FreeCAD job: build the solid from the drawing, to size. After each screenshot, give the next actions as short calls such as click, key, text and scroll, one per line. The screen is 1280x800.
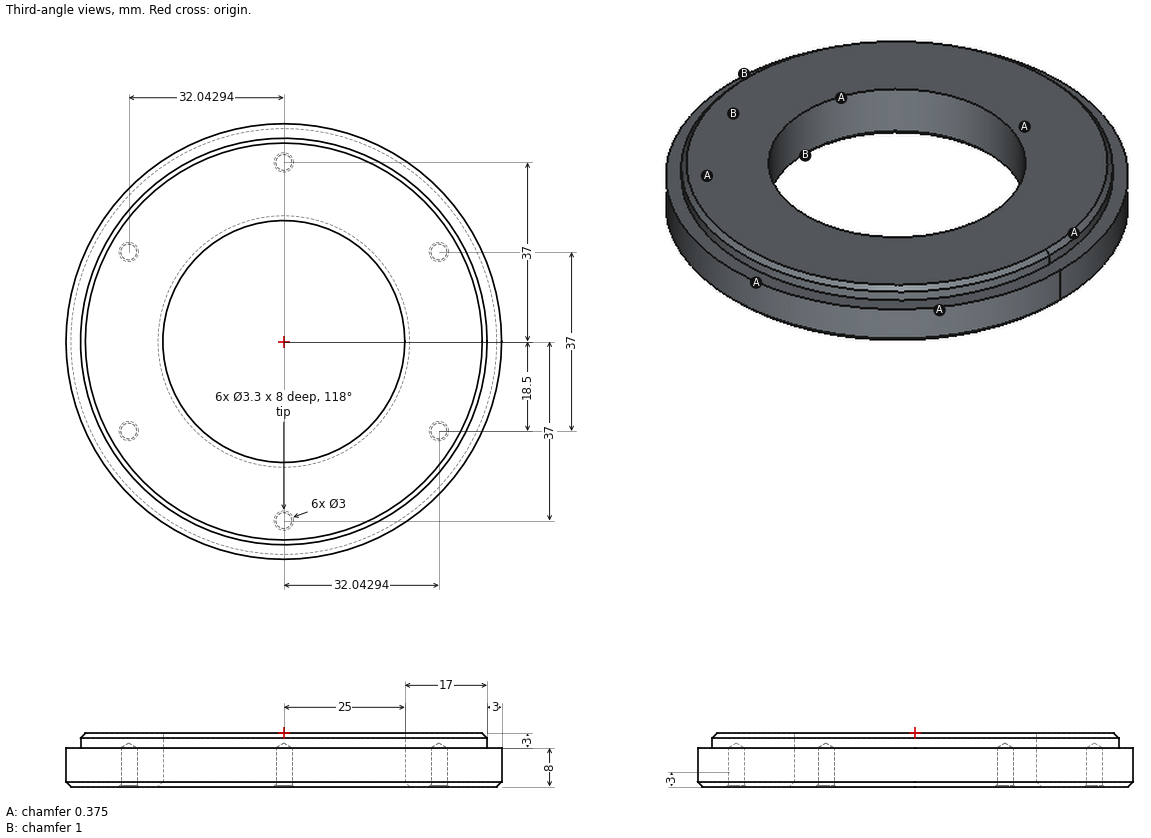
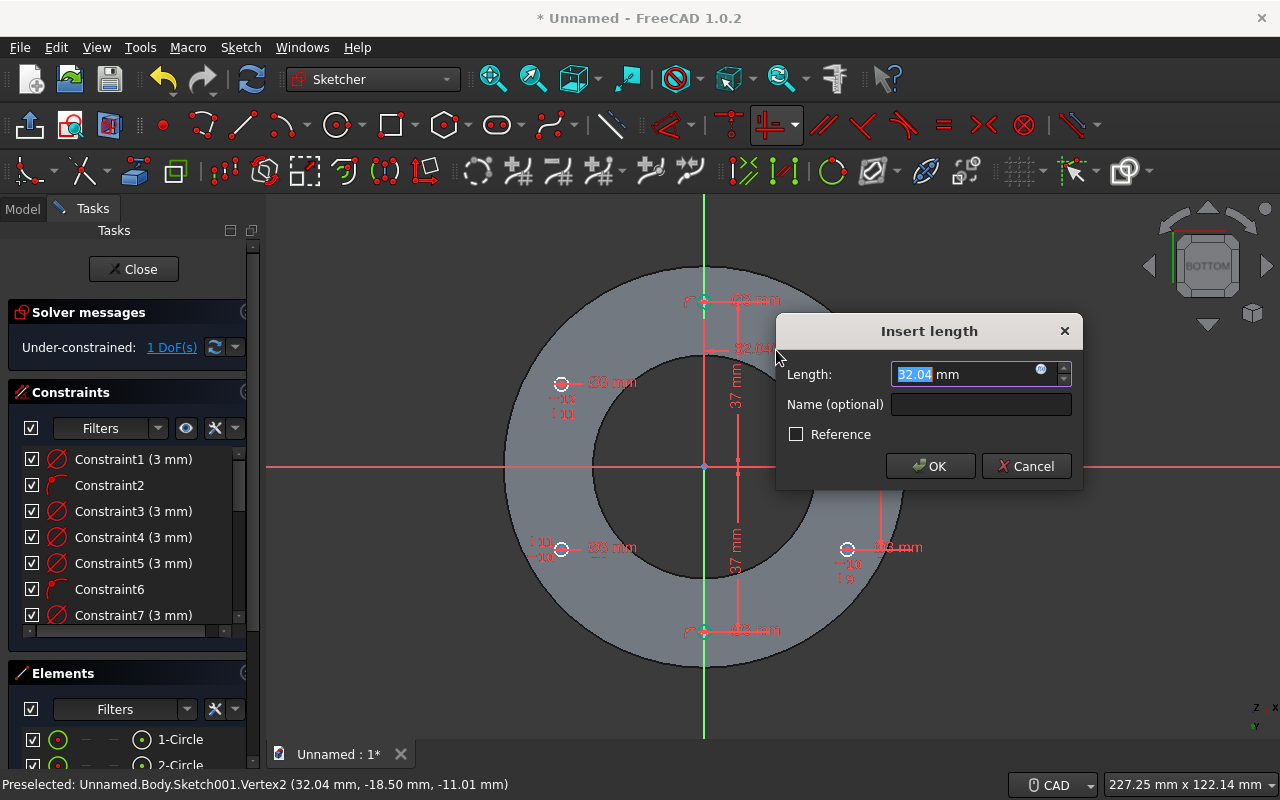
text(32.04294)
key(Return)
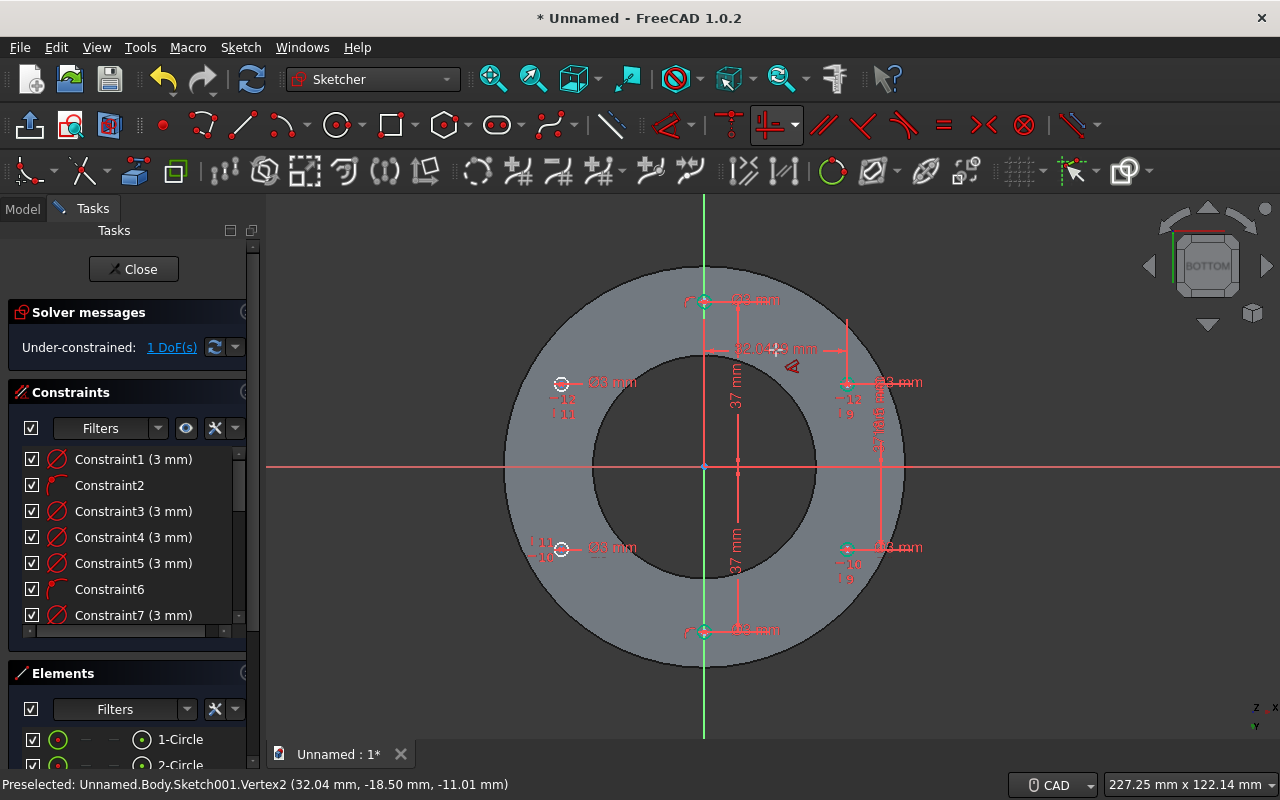
click(561, 550)
click(633, 584)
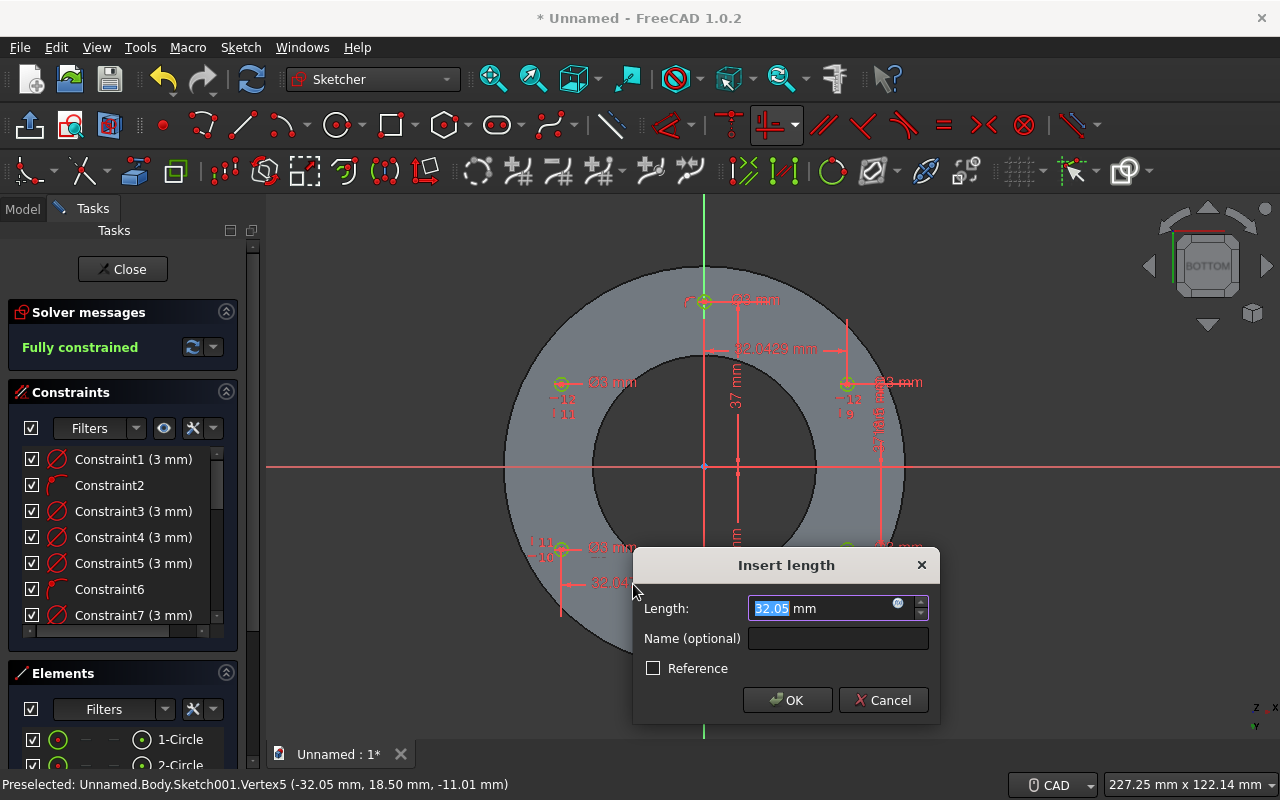
text(32.04294)
key(Return)
key(Escape)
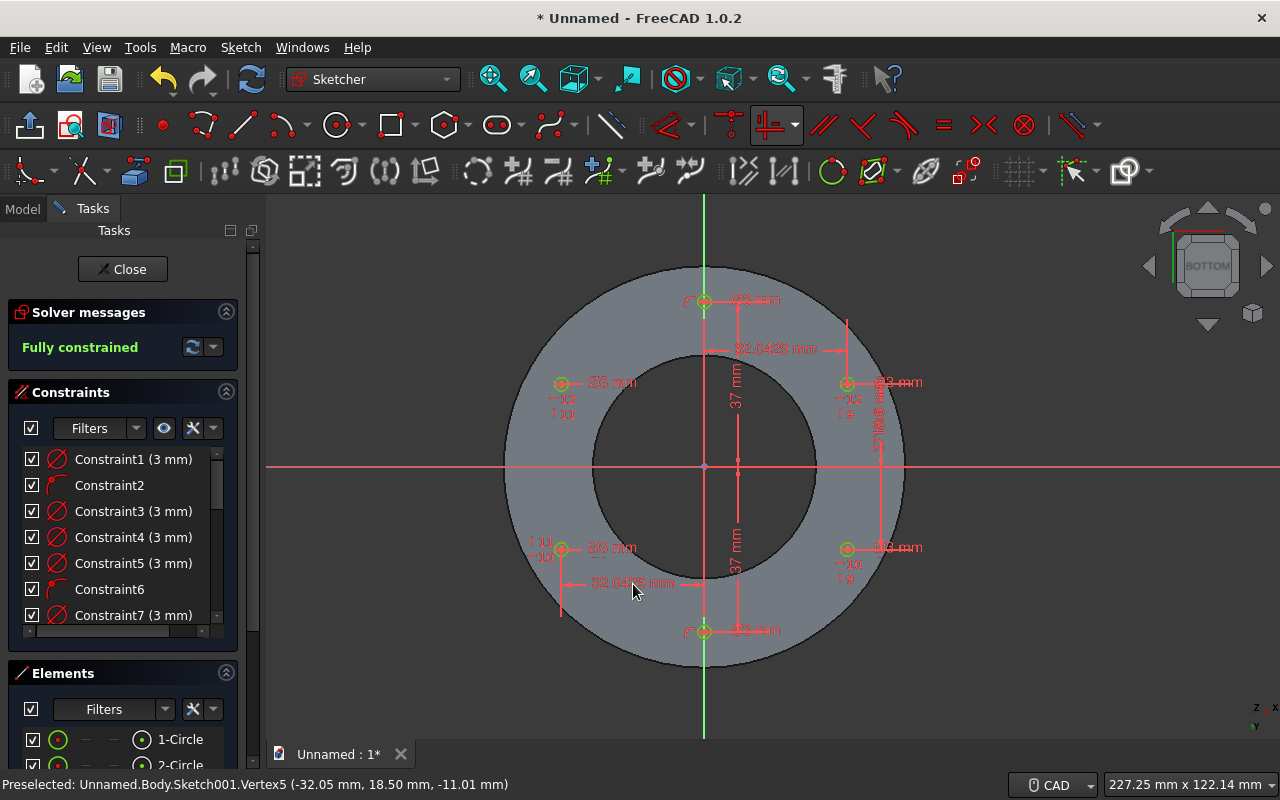
click(123, 269)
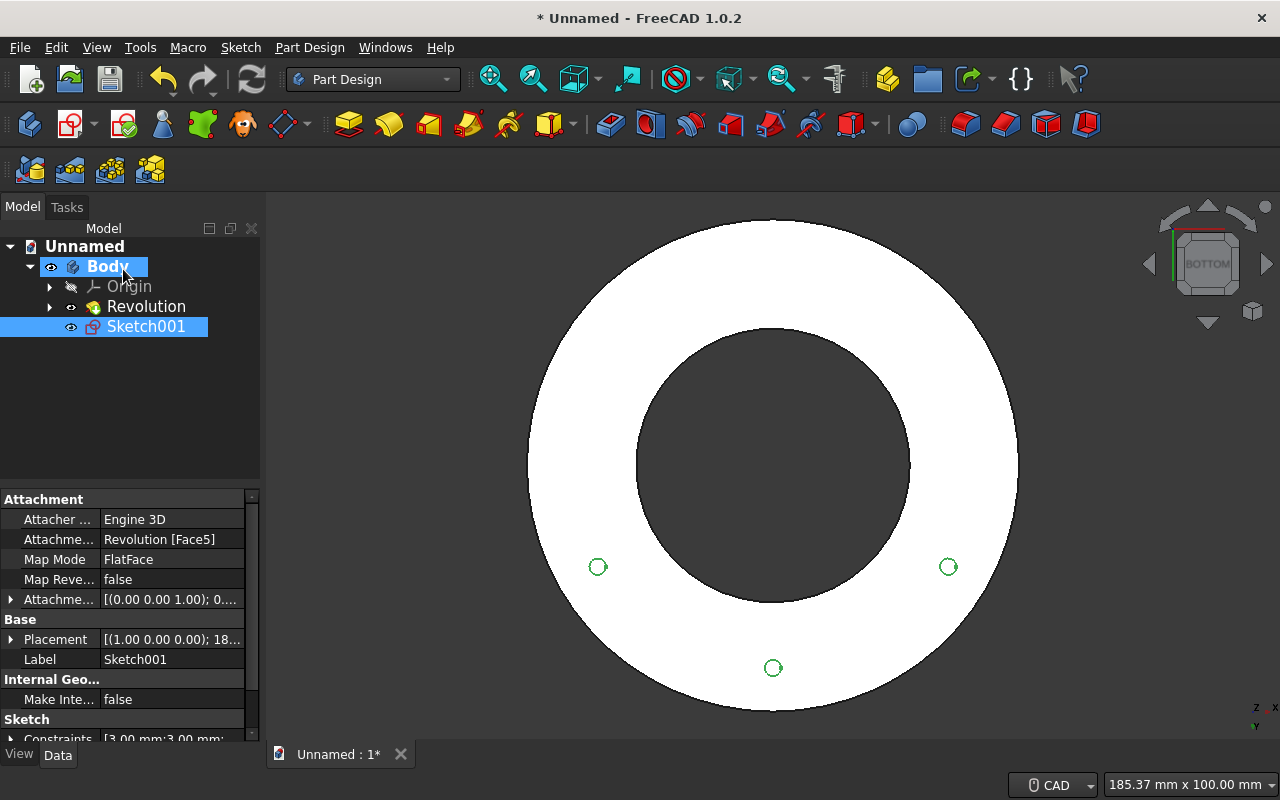
click(612, 124)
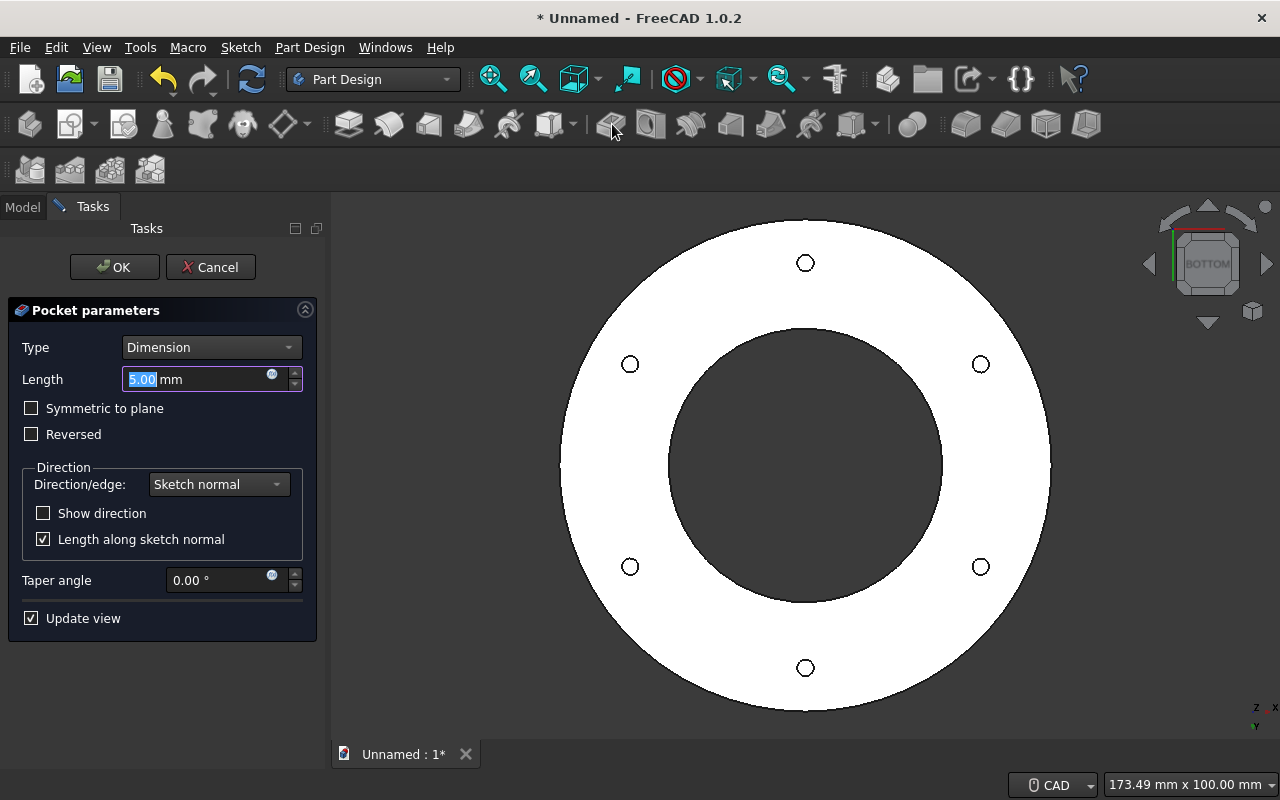
text(3)
key(Tab)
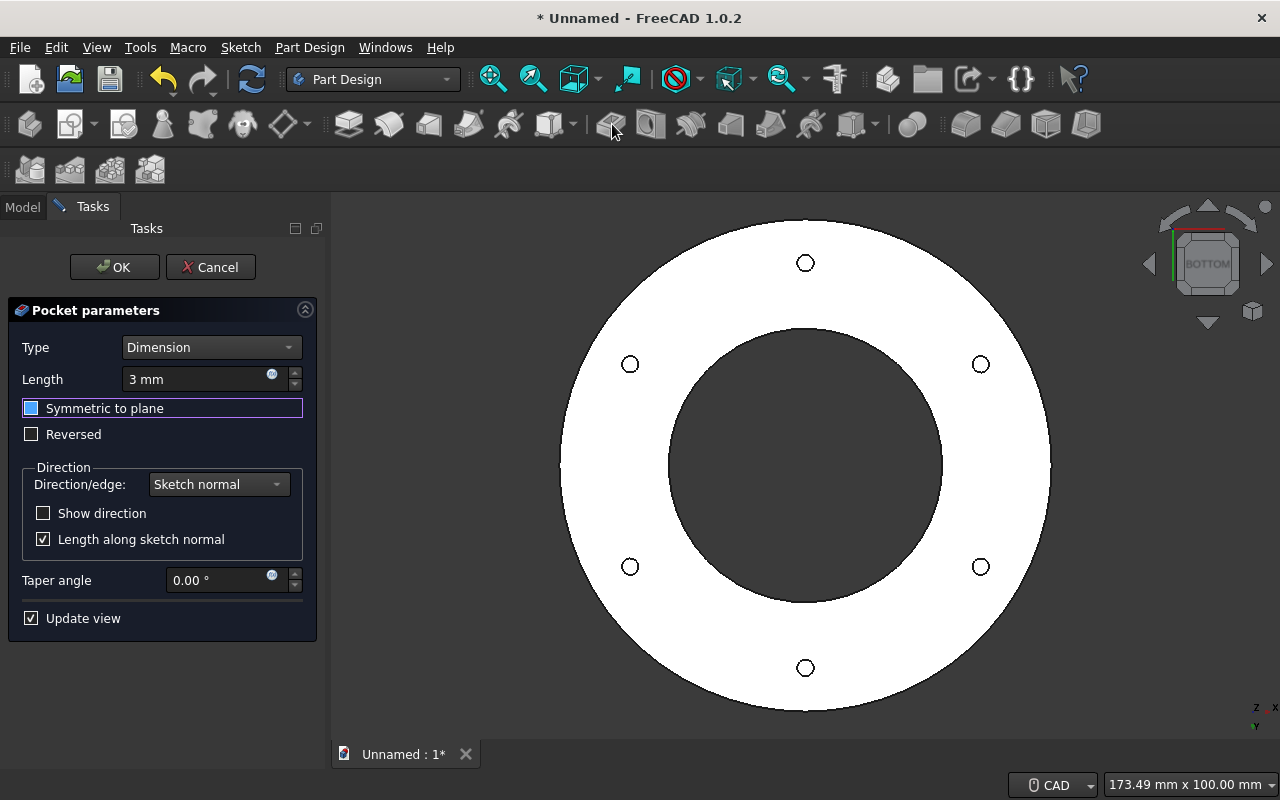
click(115, 267)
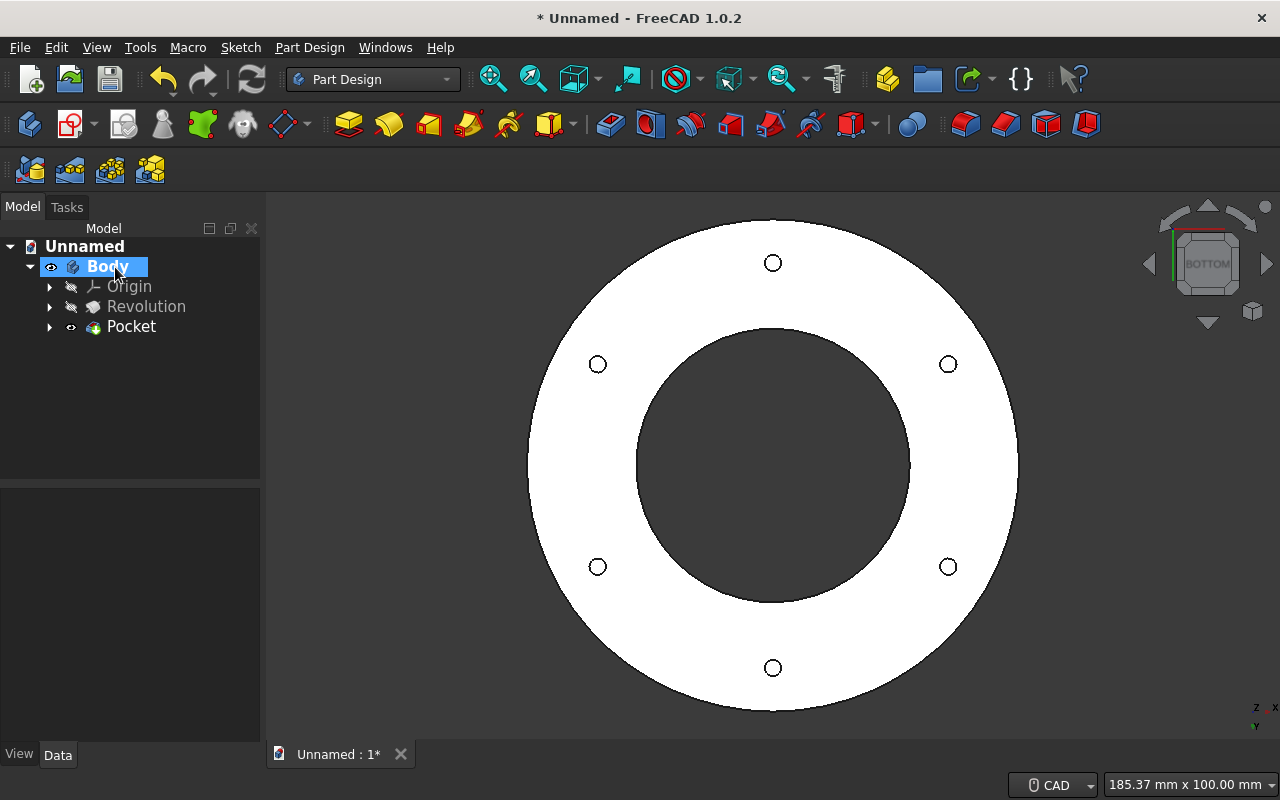
click(914, 605)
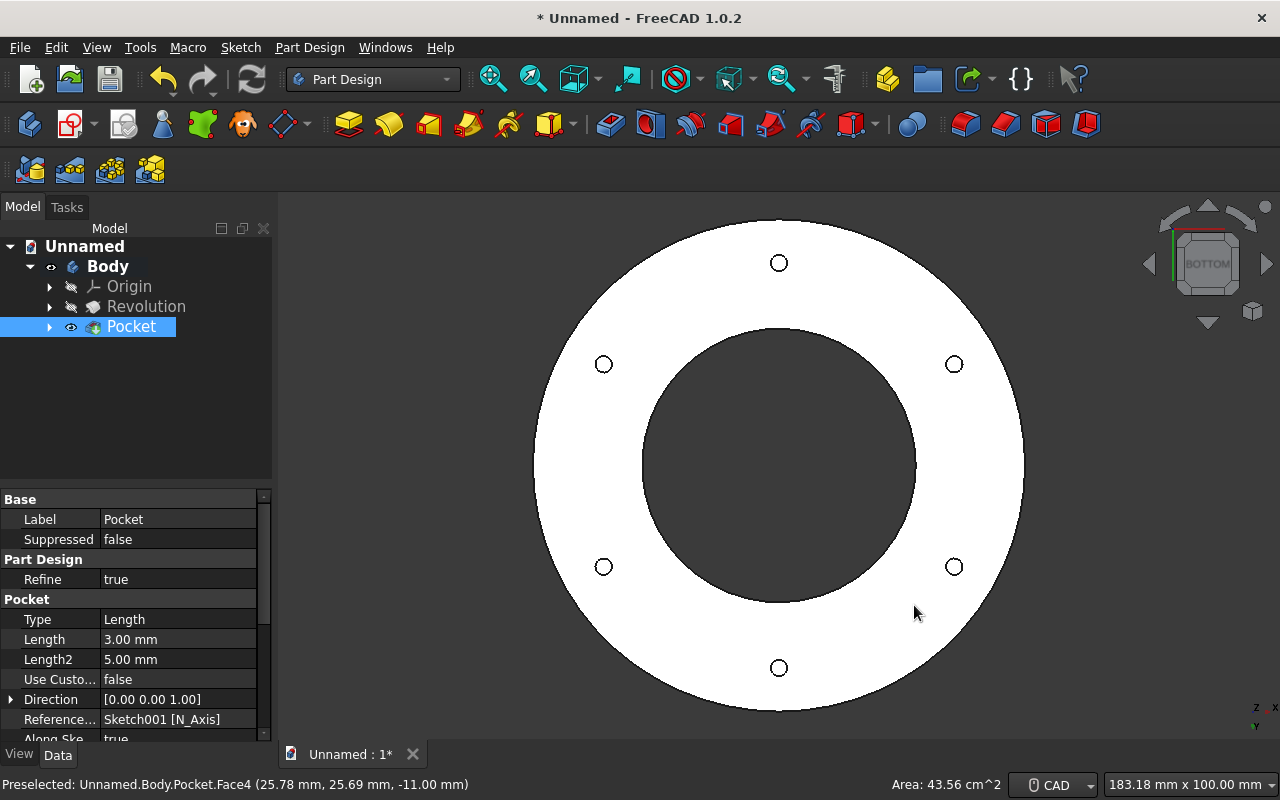
click(70, 124)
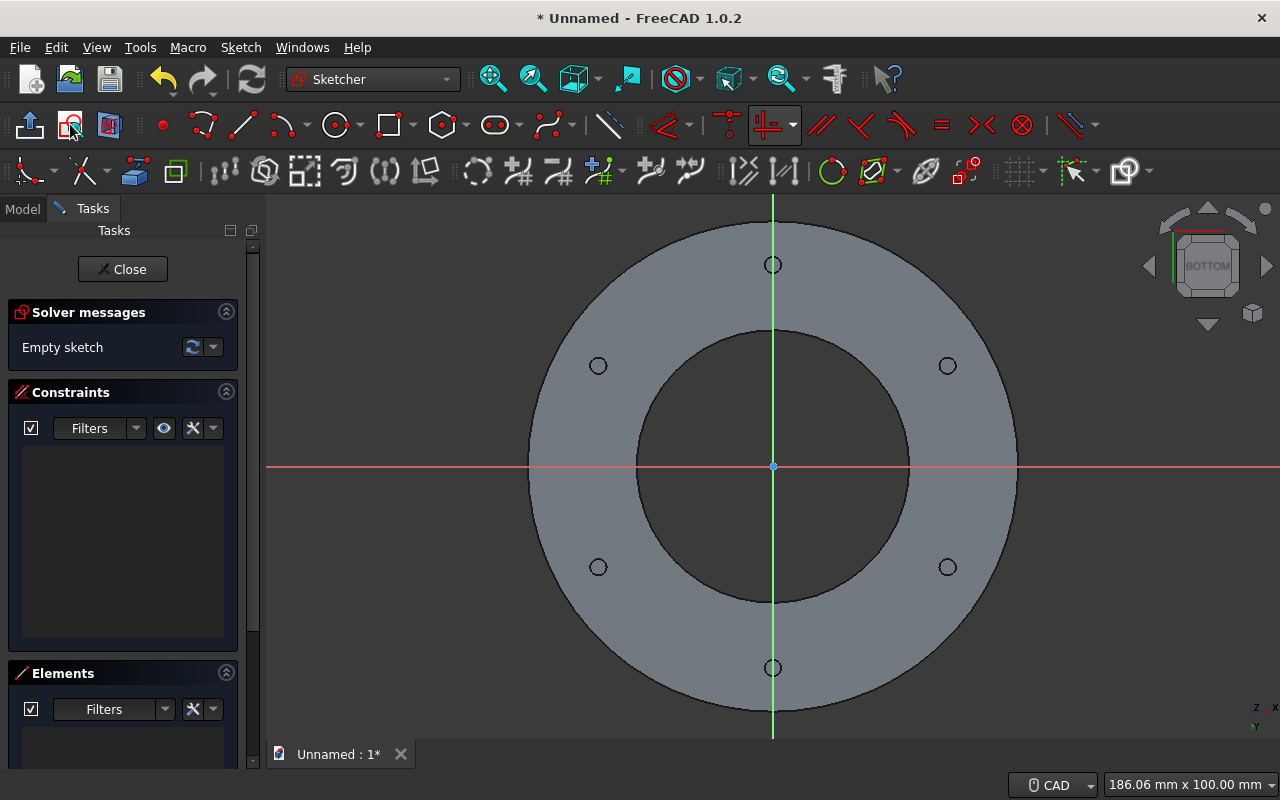
click(336, 126)